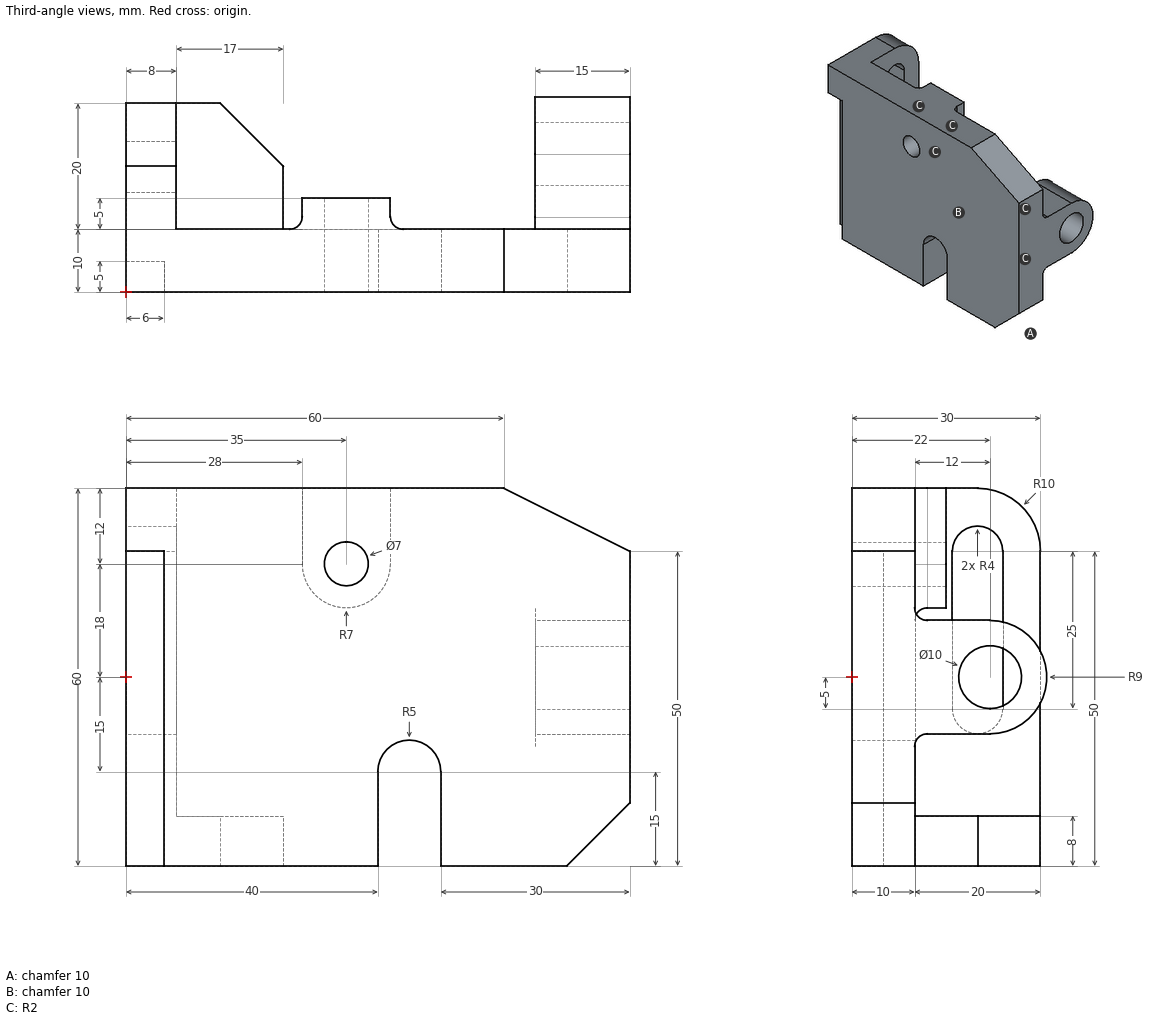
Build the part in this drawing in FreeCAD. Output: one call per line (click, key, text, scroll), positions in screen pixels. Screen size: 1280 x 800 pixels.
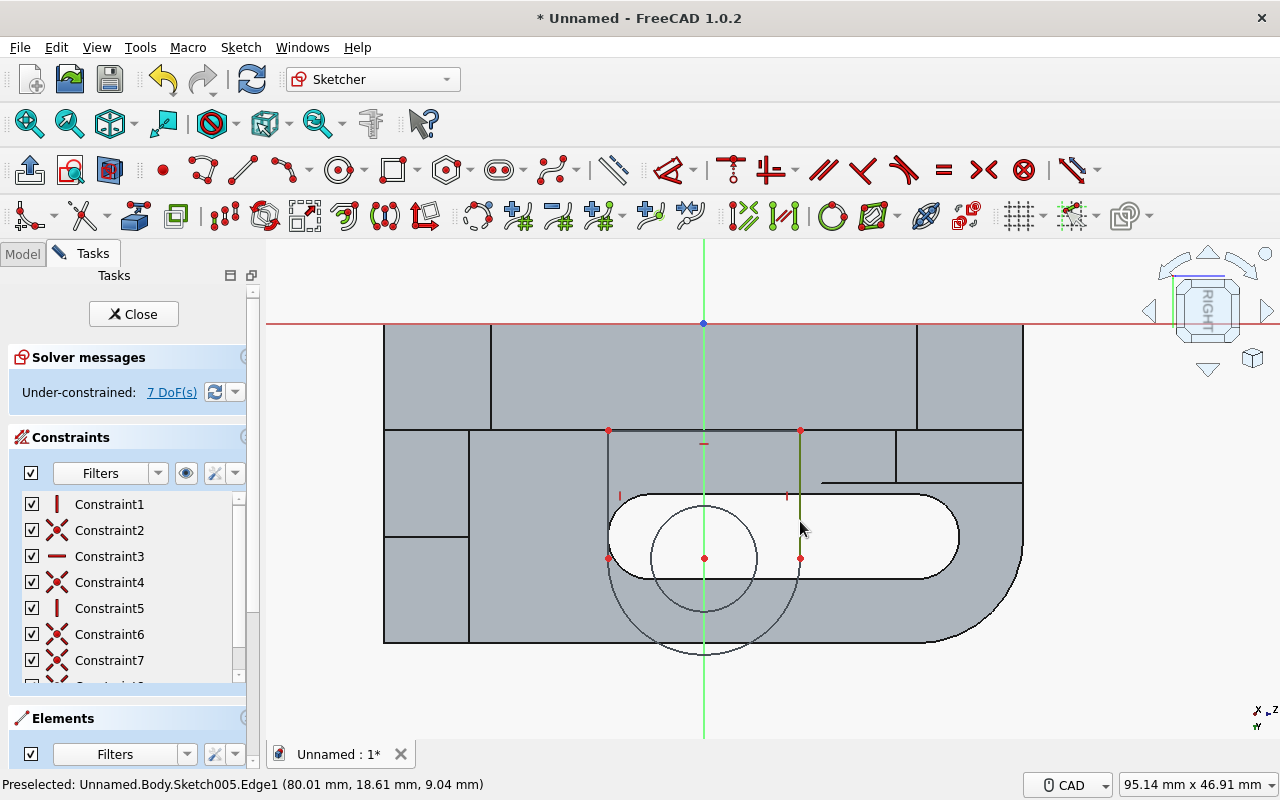
click(648, 637)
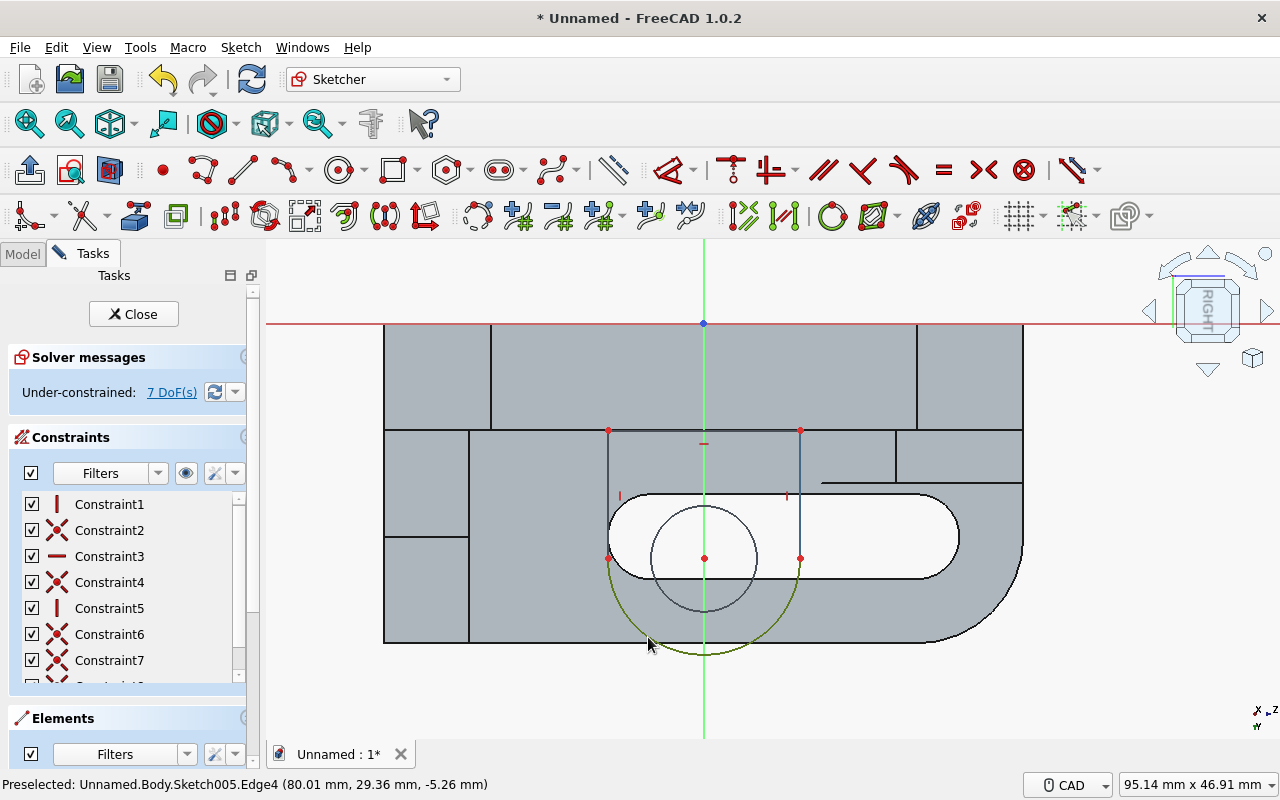
click(904, 170)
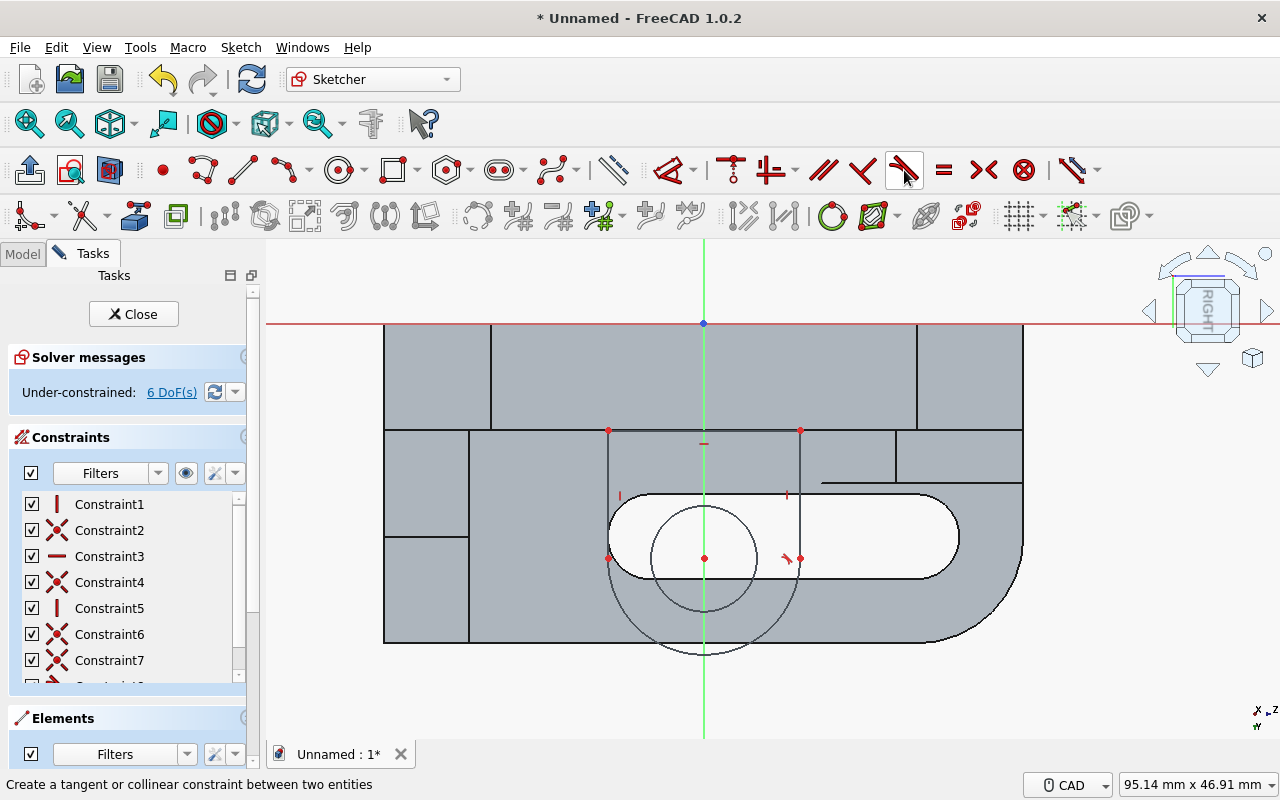
click(608, 469)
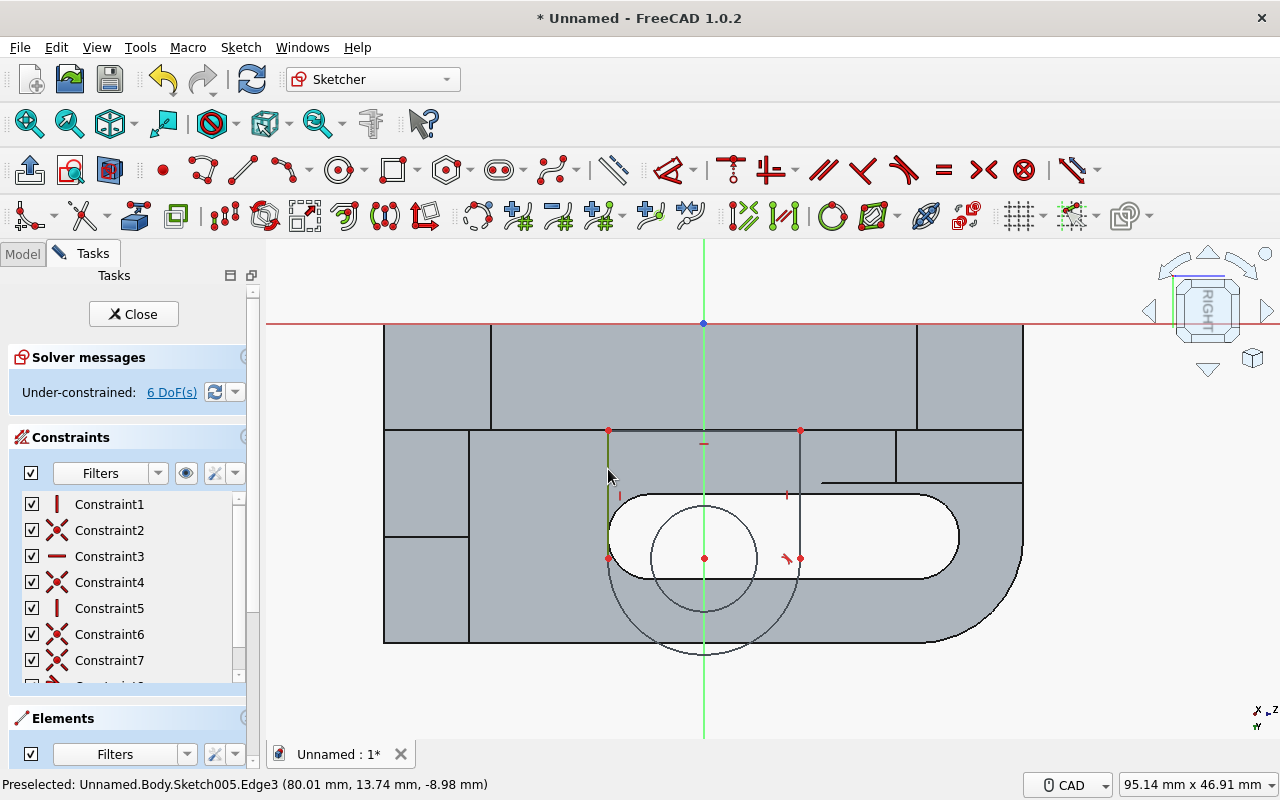
click(648, 637)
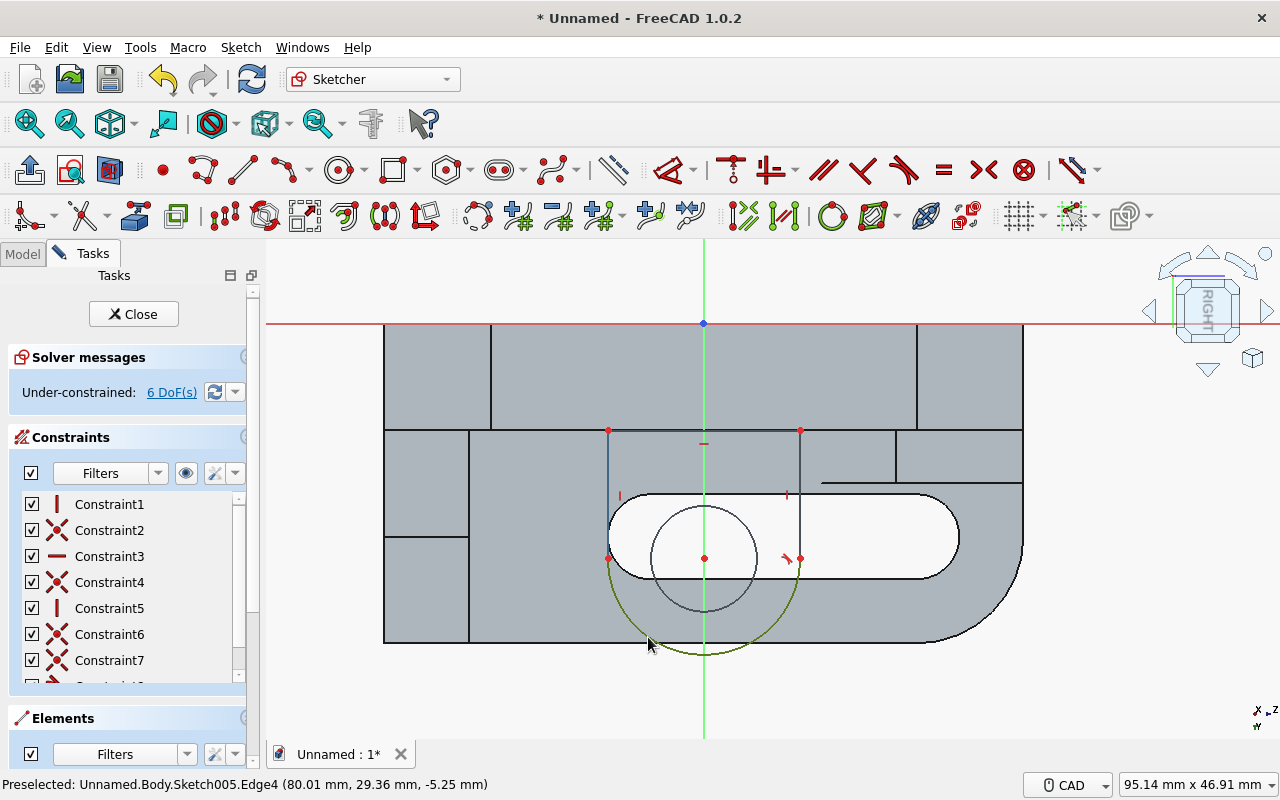
key(t)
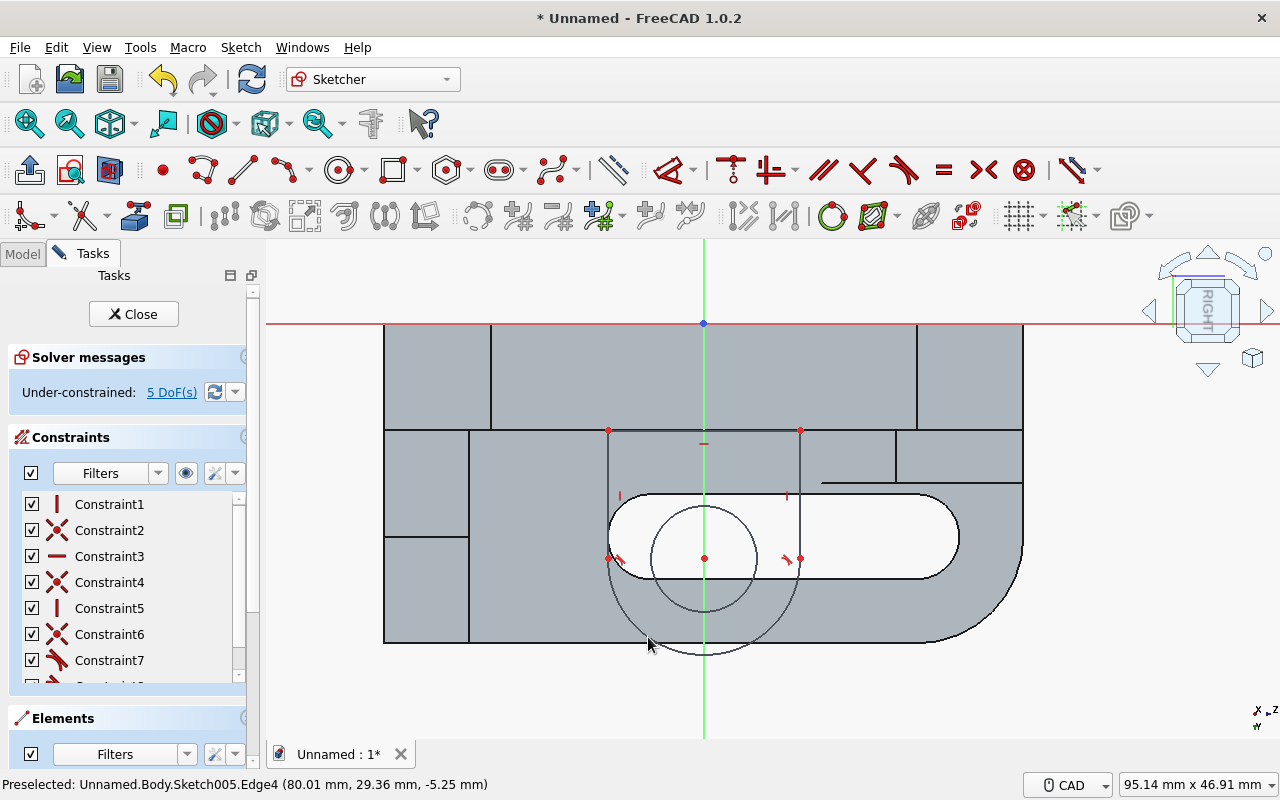
click(704, 559)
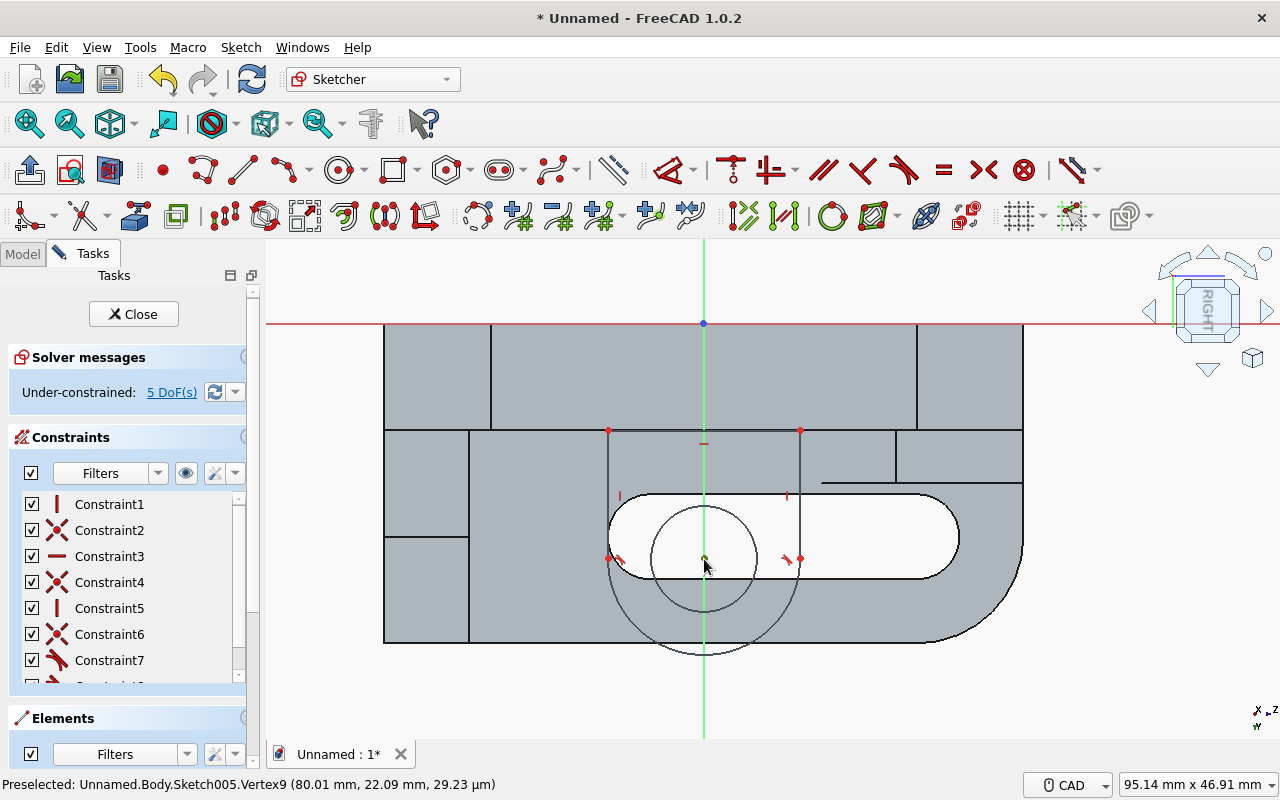
click(704, 552)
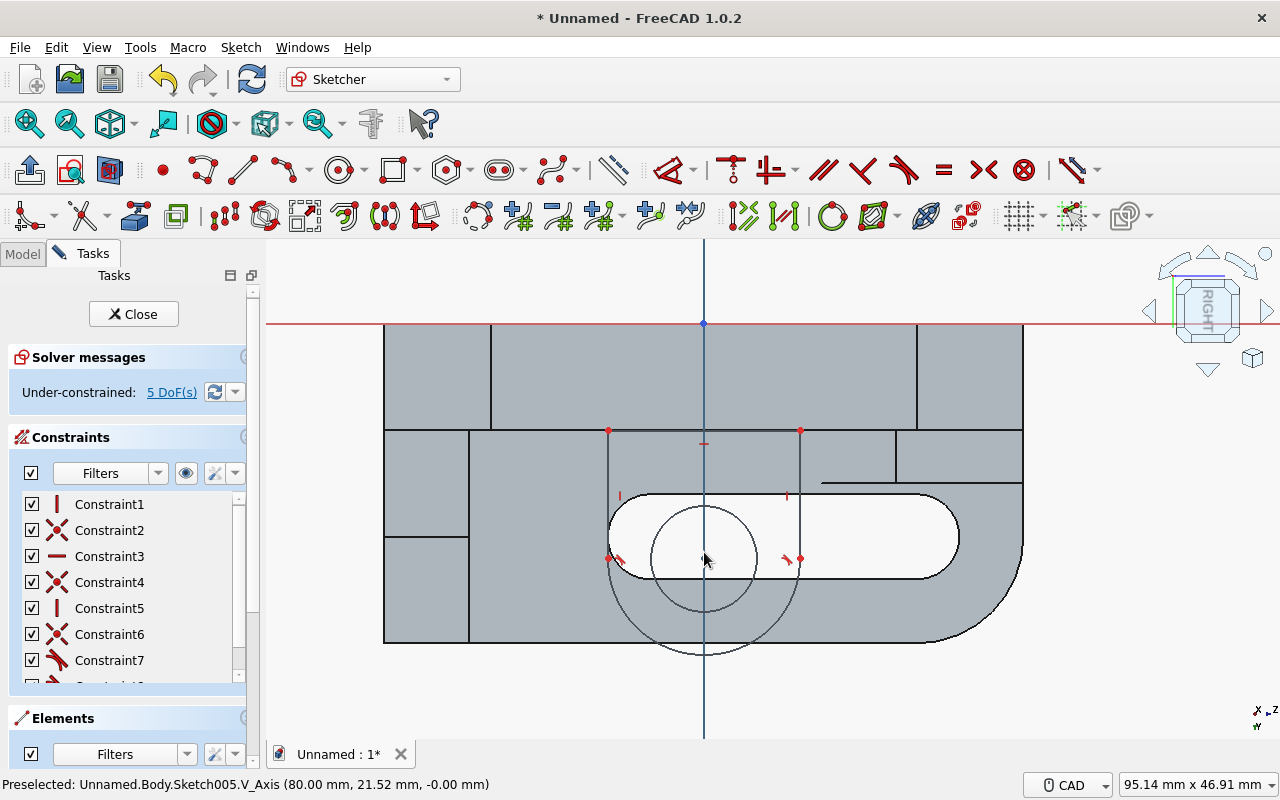
key(c)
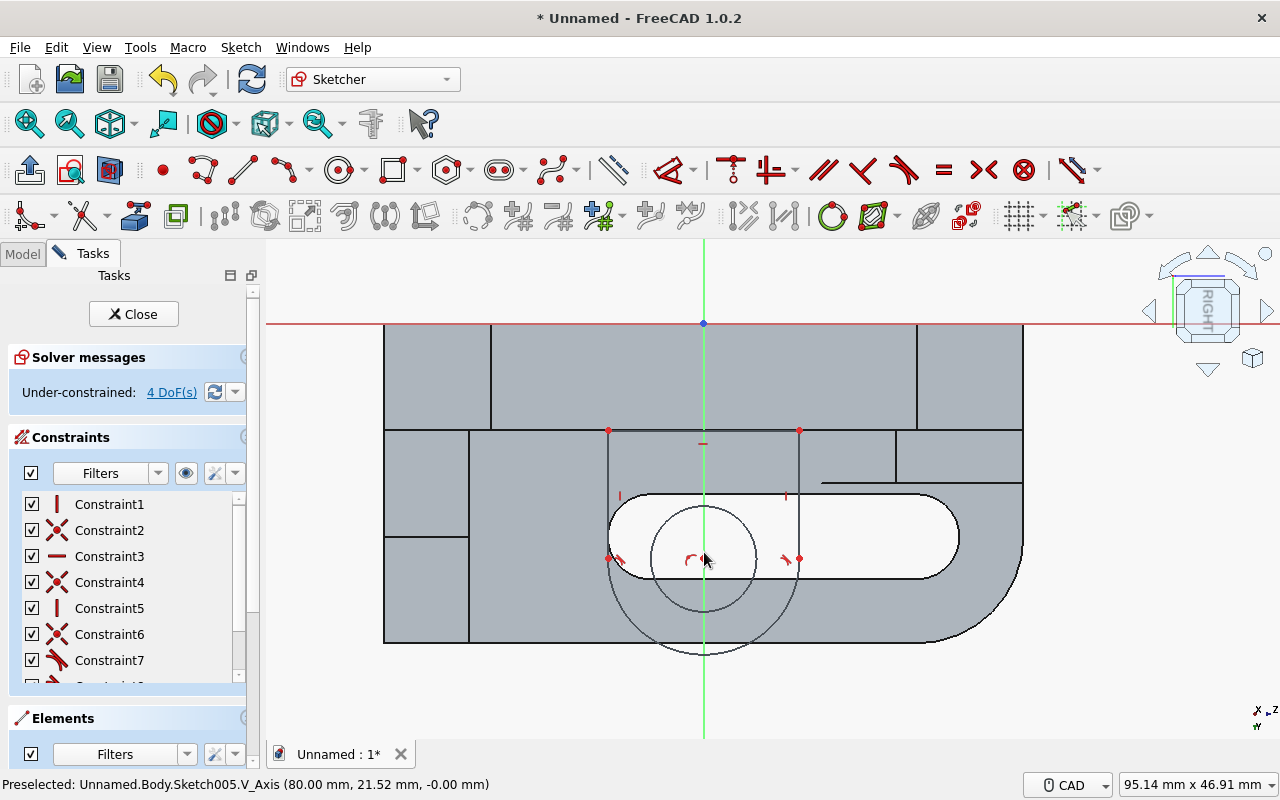
click(668, 170)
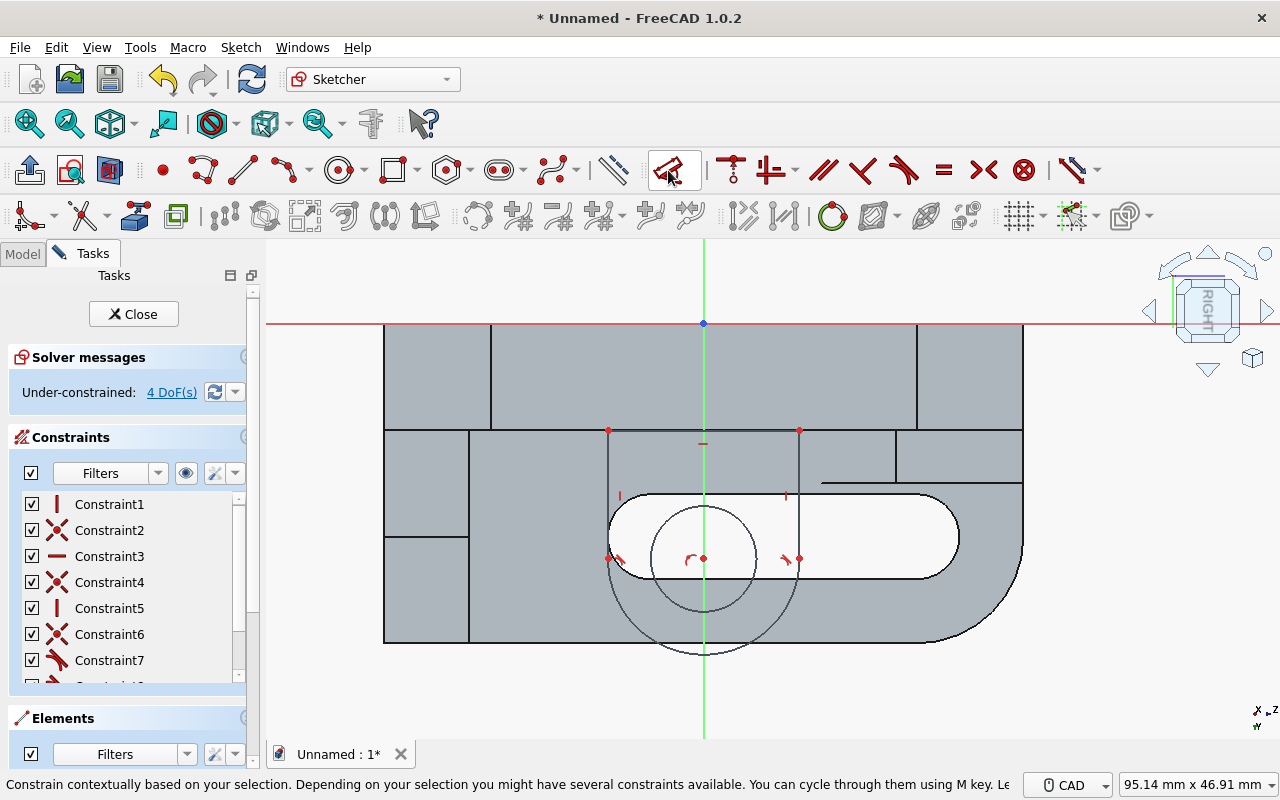
click(647, 636)
click(628, 662)